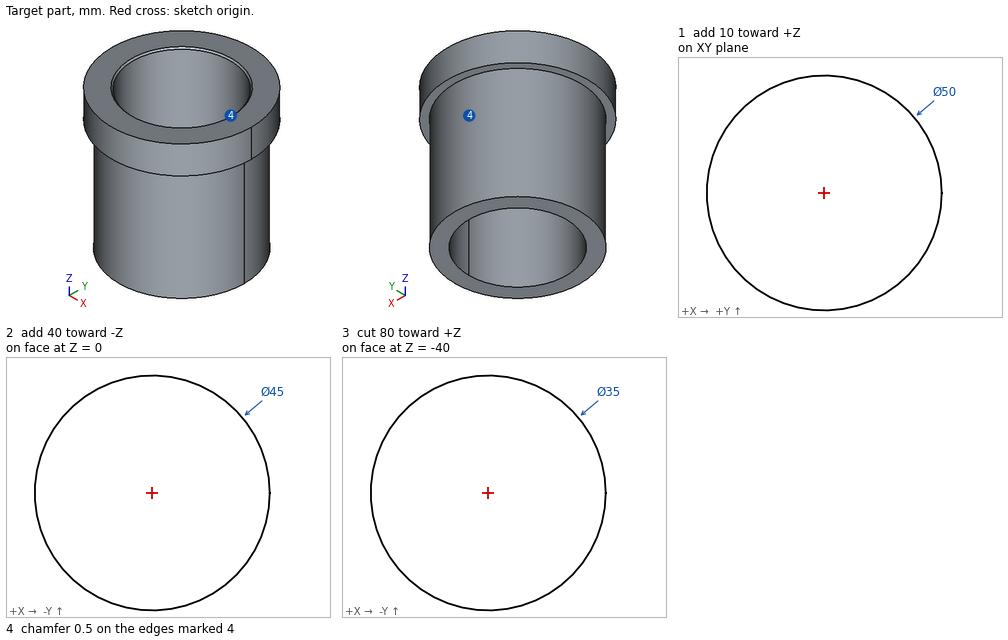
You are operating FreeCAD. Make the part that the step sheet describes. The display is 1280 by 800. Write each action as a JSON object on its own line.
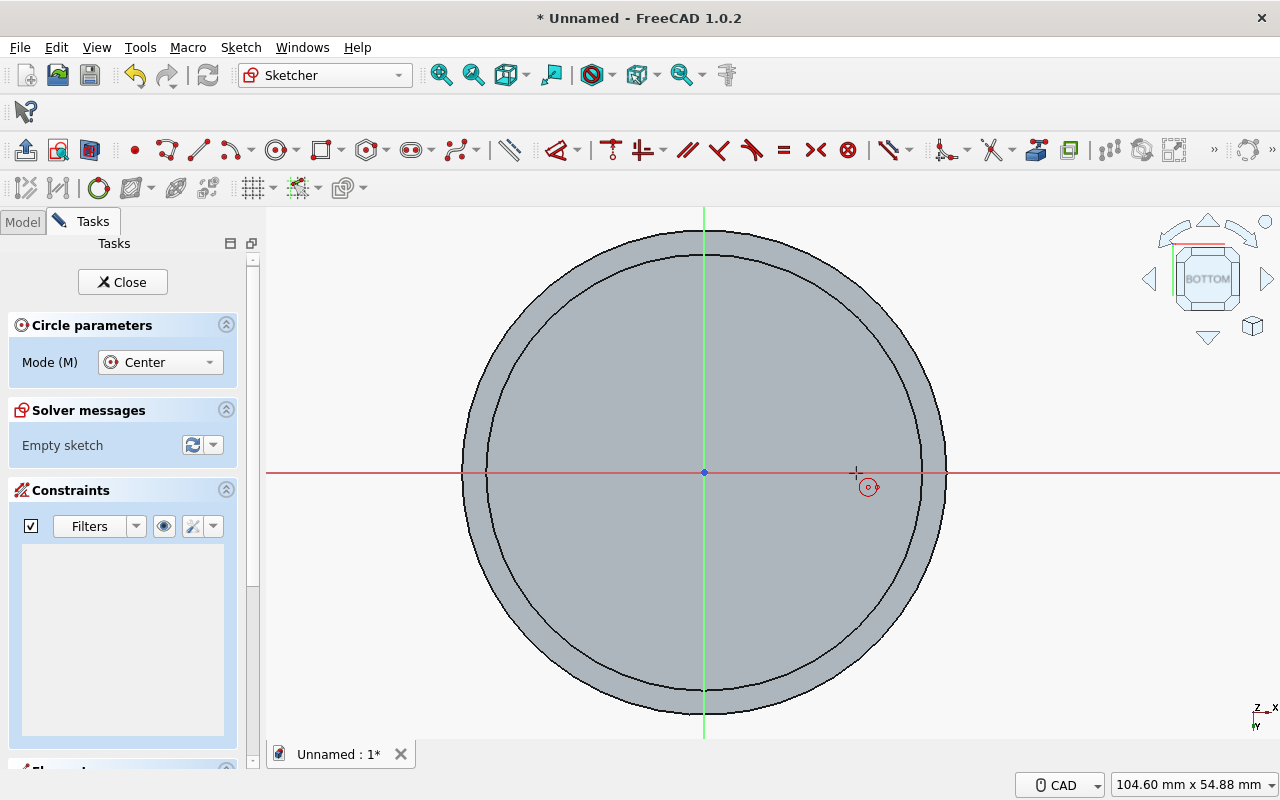
{"action": "left_click", "coordinate": [704, 473]}
{"action": "left_click", "coordinate": [824, 353]}
{"action": "key", "text": "Escape"}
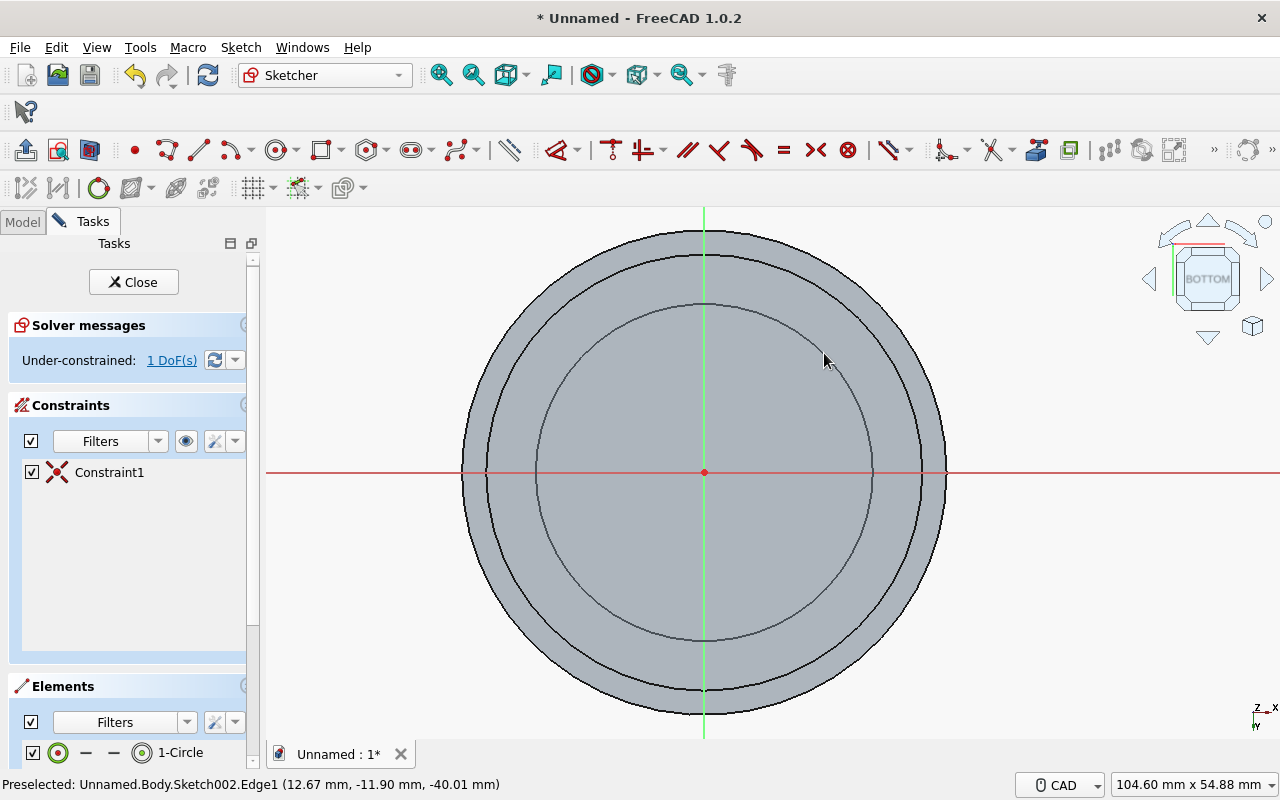
{"action": "left_click", "coordinate": [556, 150]}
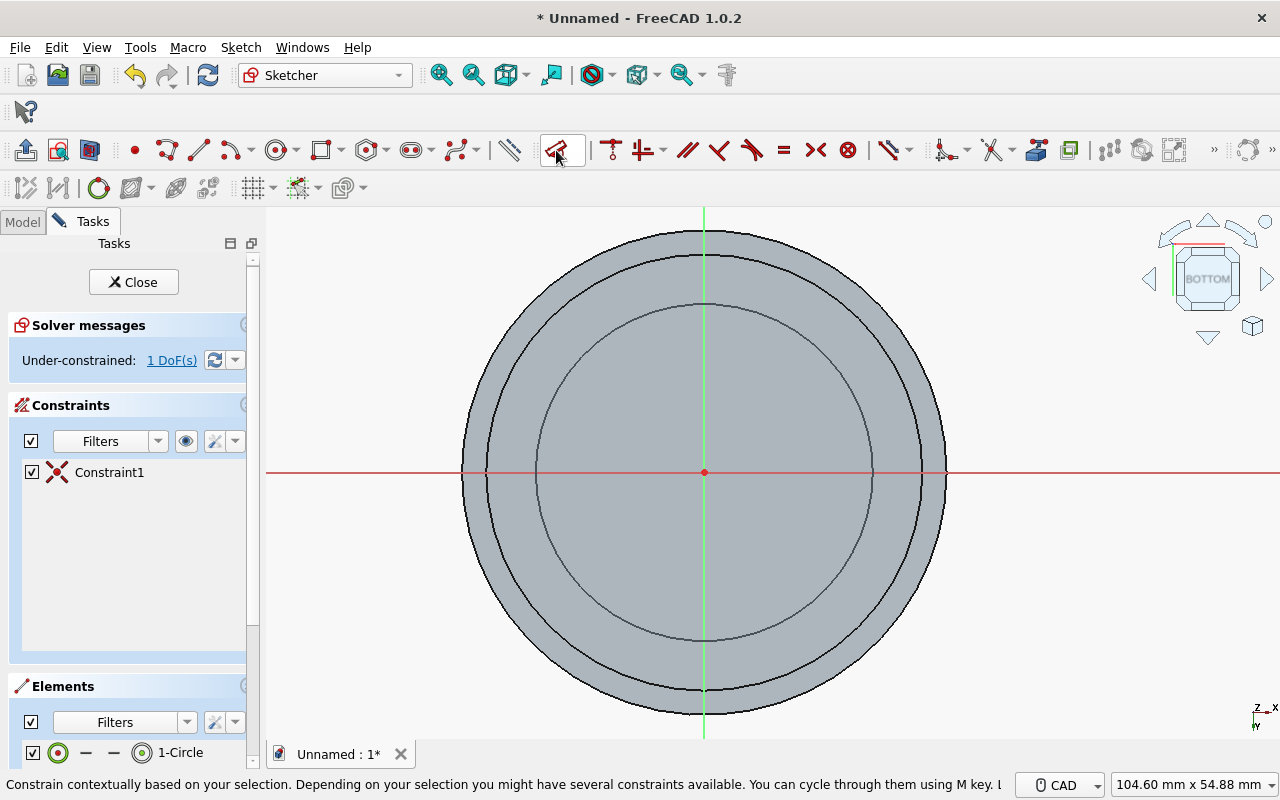
{"action": "left_click", "coordinate": [823, 353]}
{"action": "left_click", "coordinate": [846, 330]}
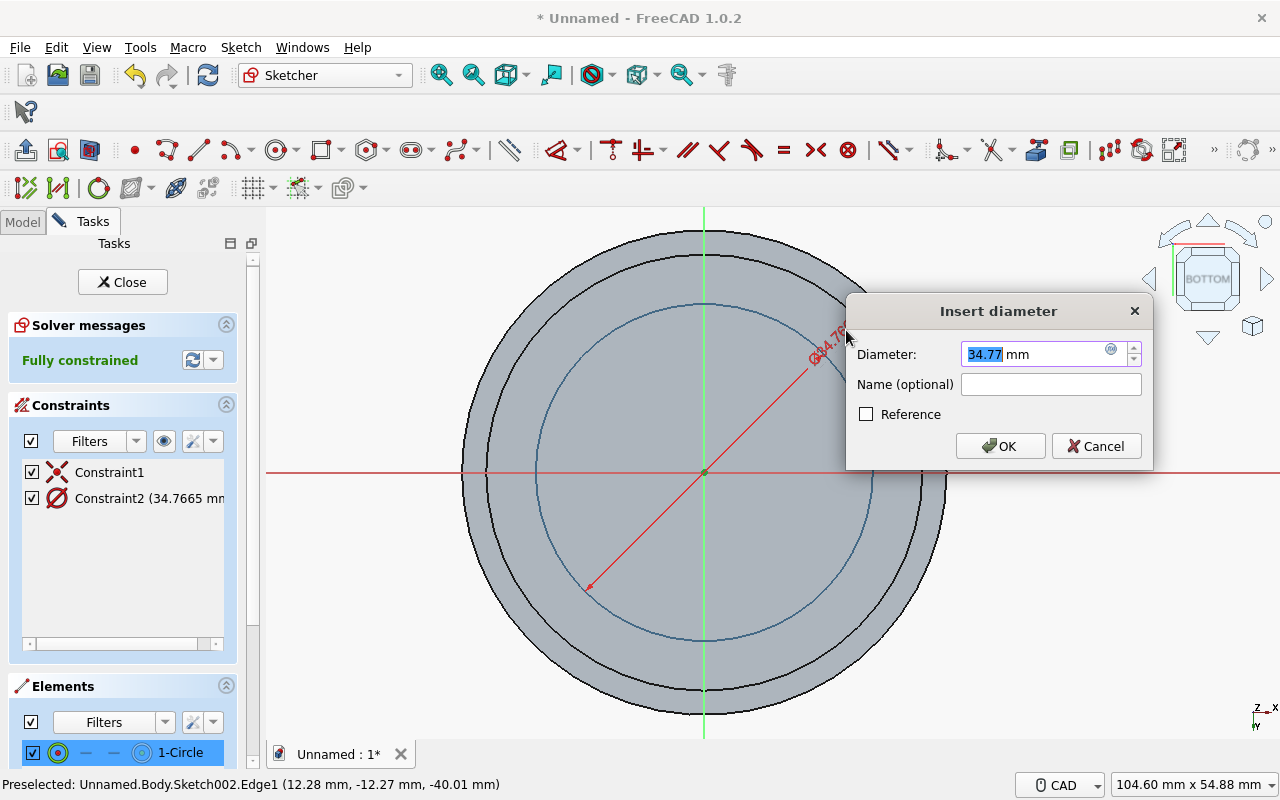
{"action": "type", "text": "35"}
{"action": "key", "text": "Return"}
{"action": "key", "text": "Escape"}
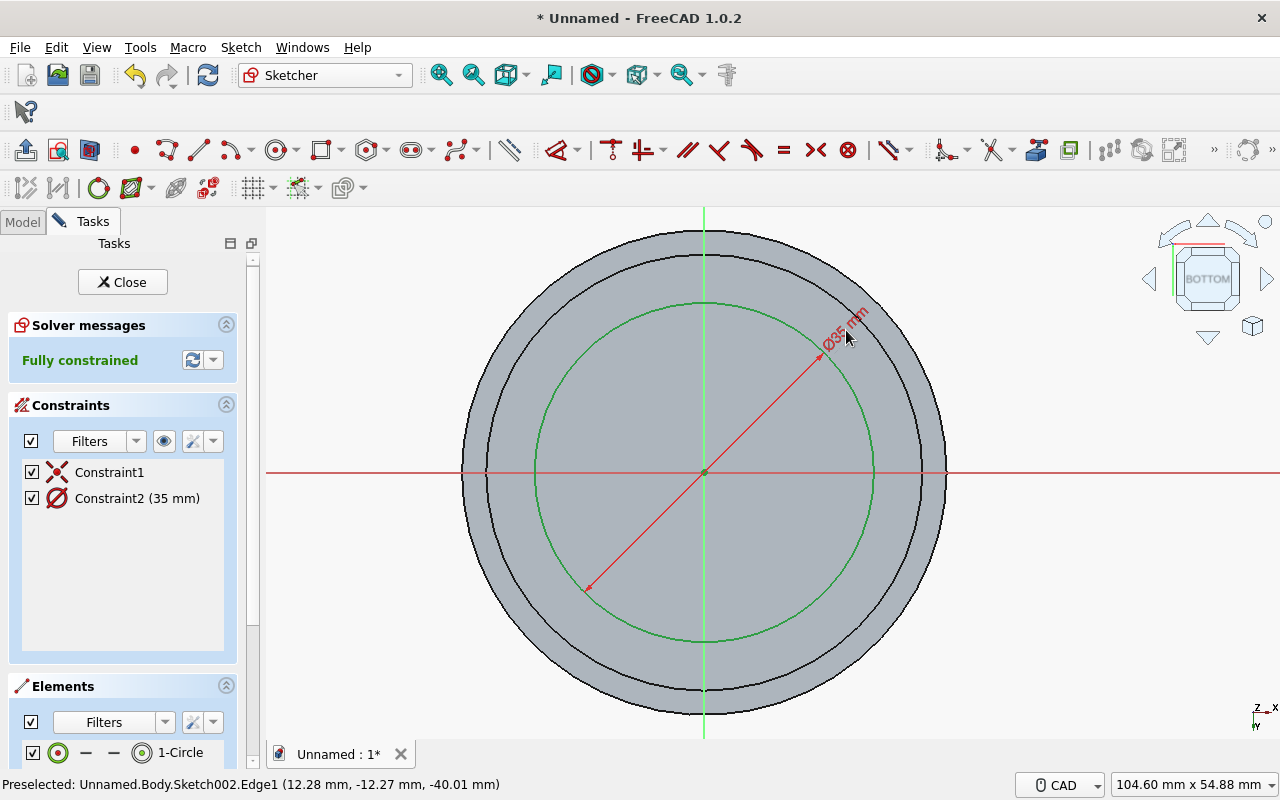
{"action": "left_click", "coordinate": [123, 282]}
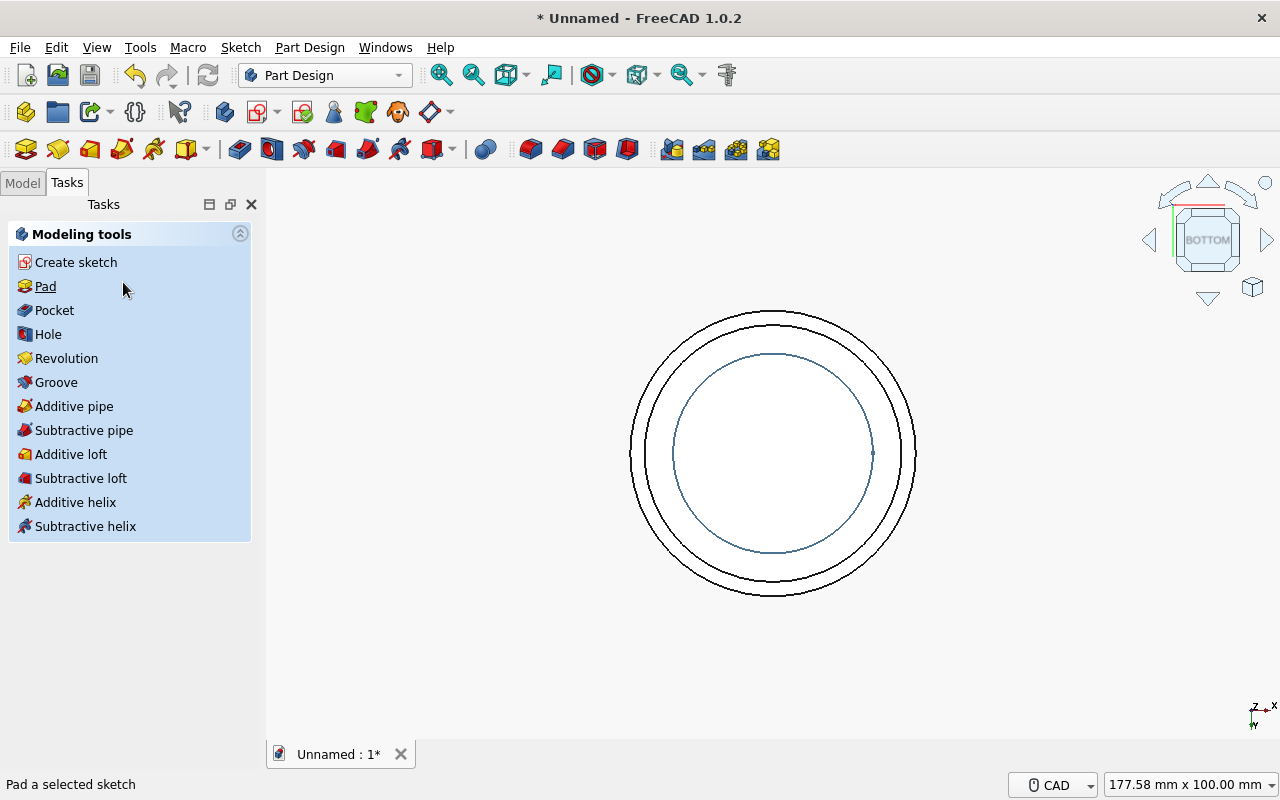
{"action": "left_click", "coordinate": [240, 150]}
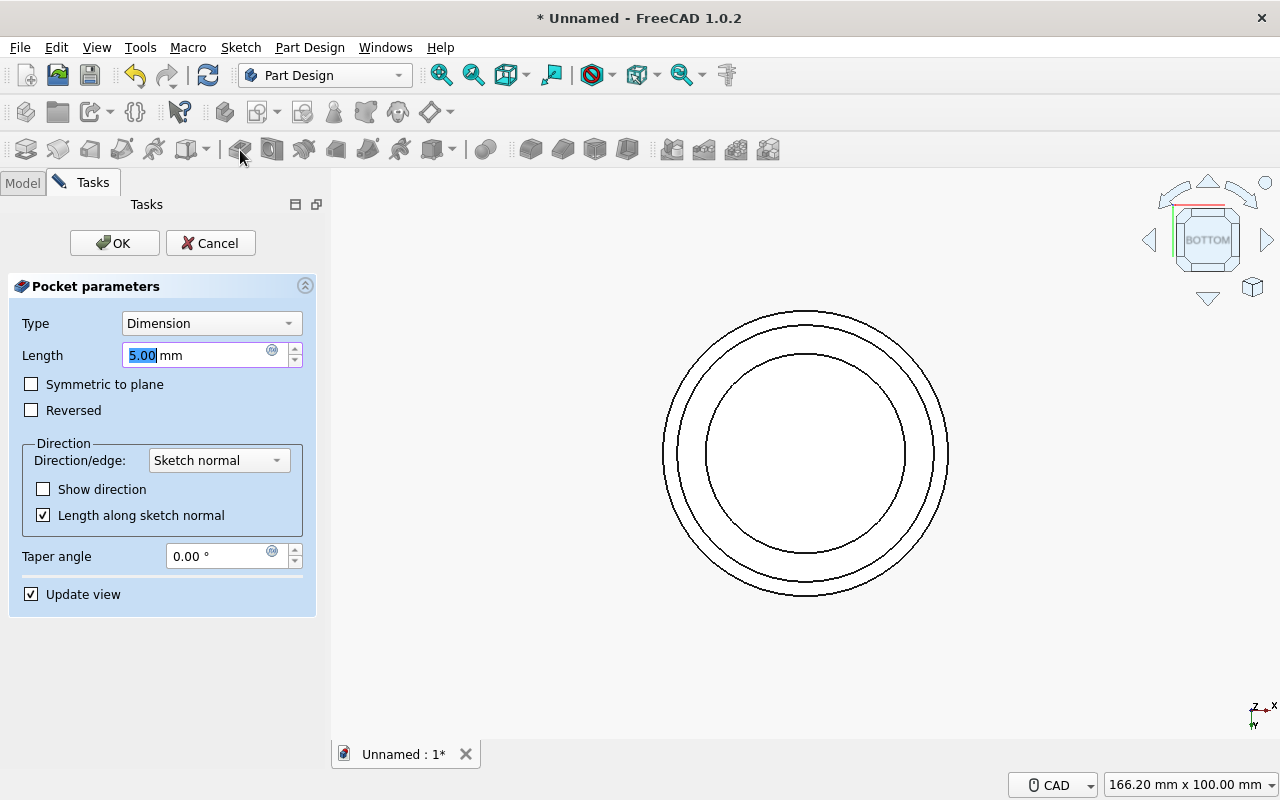
{"action": "type", "text": "80"}
{"action": "key", "text": "Tab"}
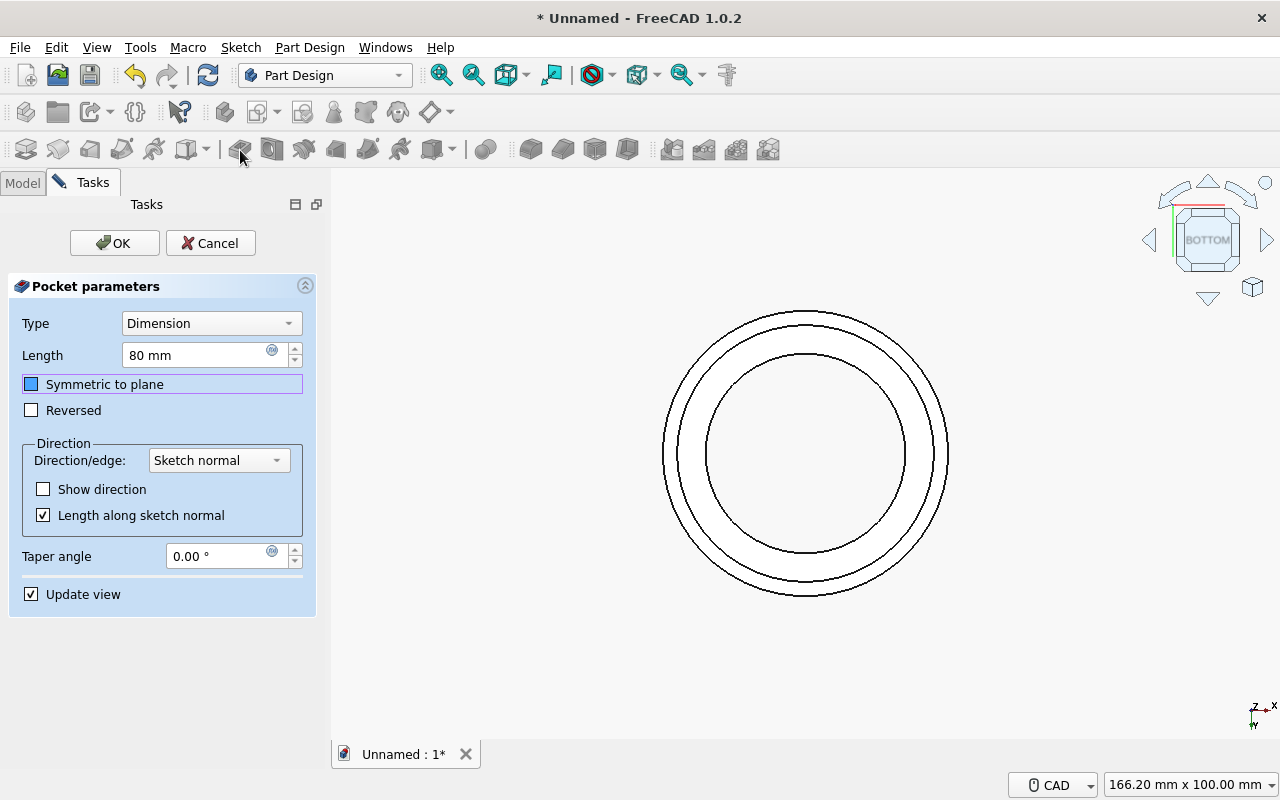
{"action": "left_click", "coordinate": [115, 243]}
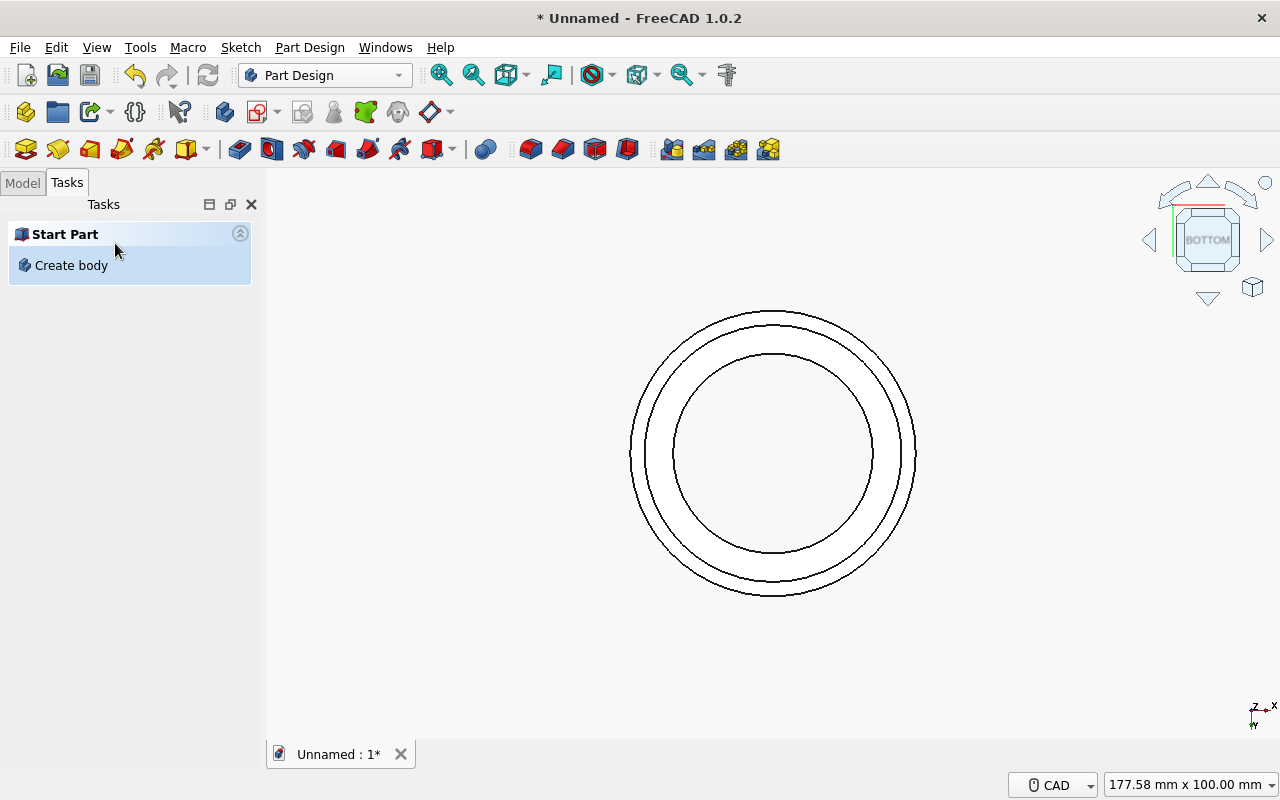
{"action": "key", "text": "0"}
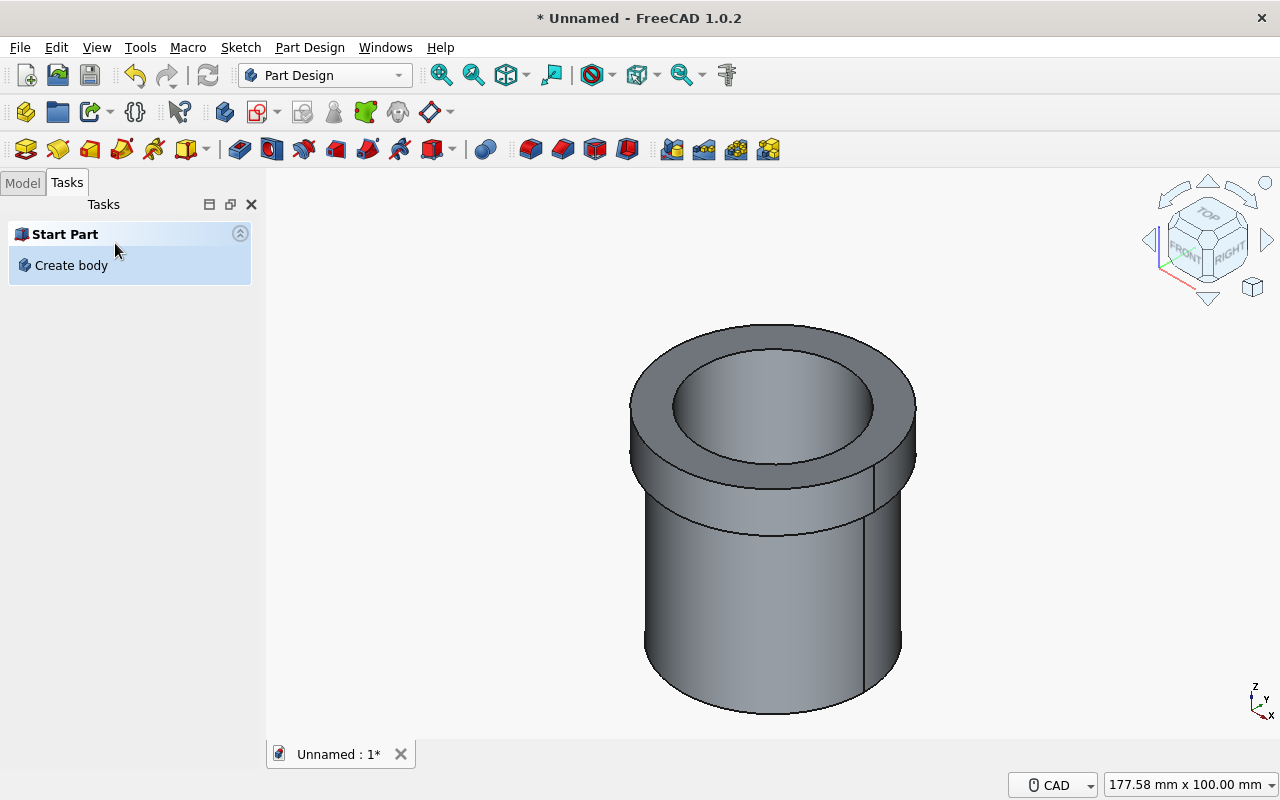
{"action": "key", "text": "v f"}